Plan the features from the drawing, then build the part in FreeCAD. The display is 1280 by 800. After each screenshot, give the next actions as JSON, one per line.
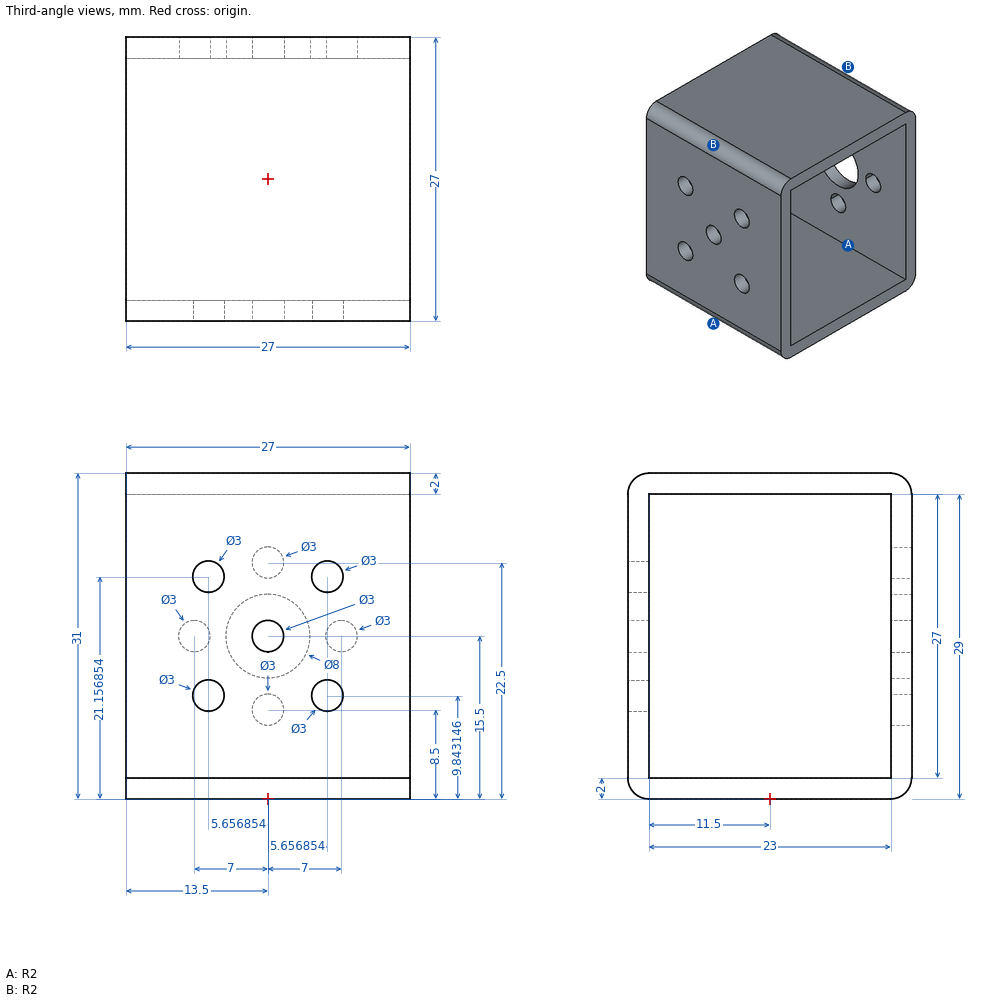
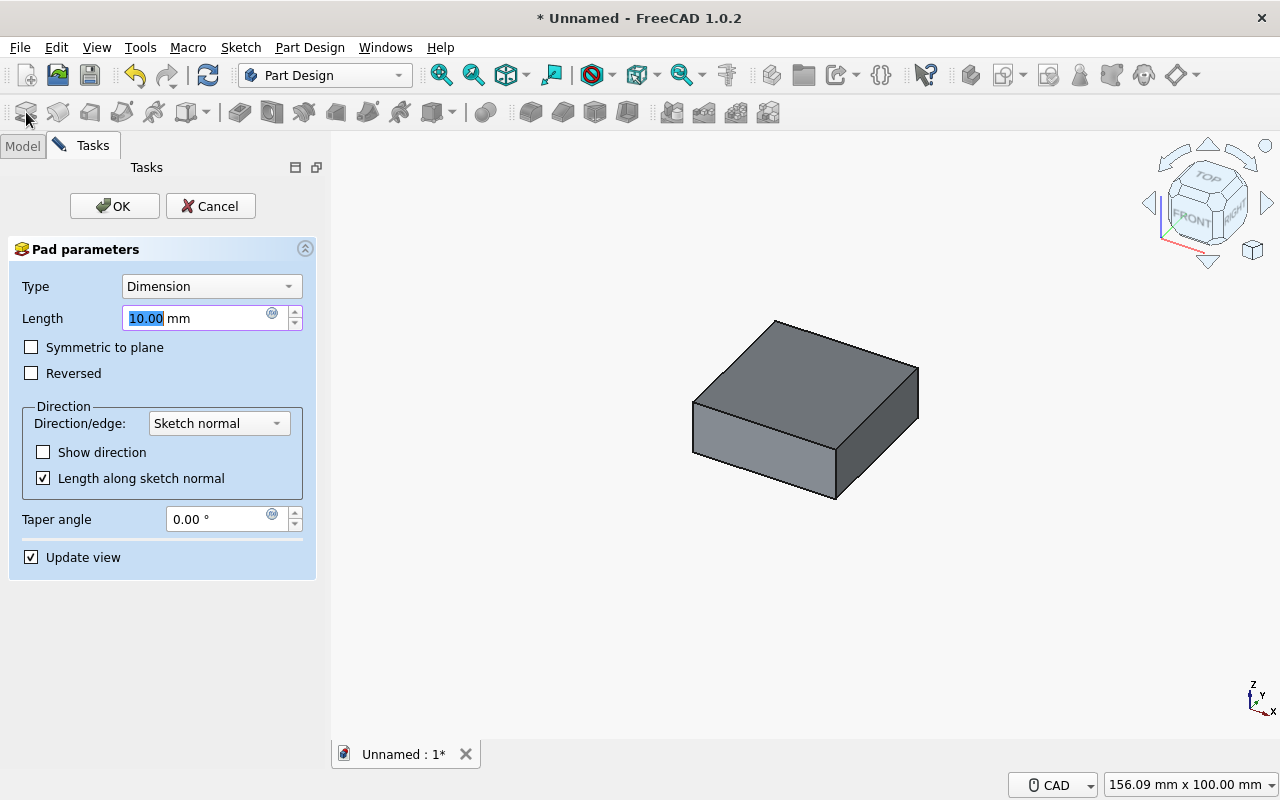
{"action": "type", "text": "29"}
{"action": "key", "text": "Tab"}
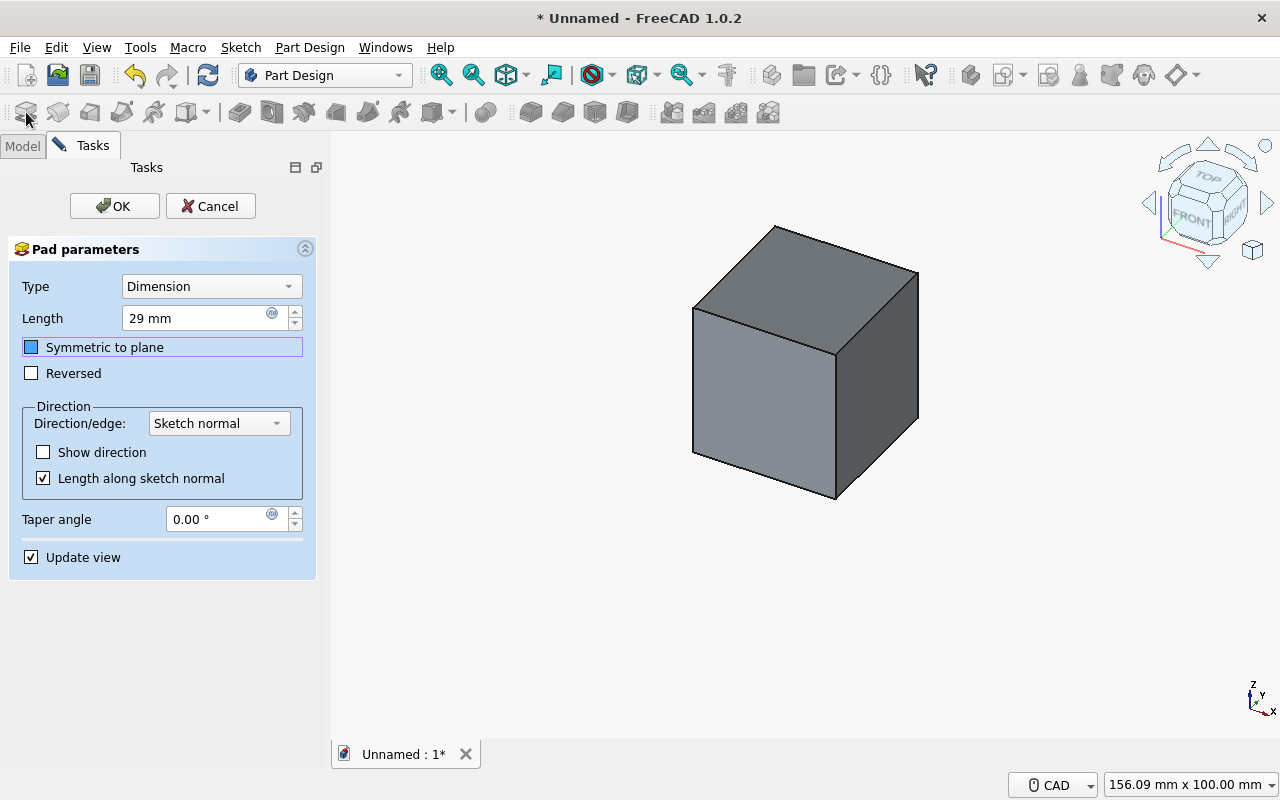
{"action": "left_click", "coordinate": [115, 206]}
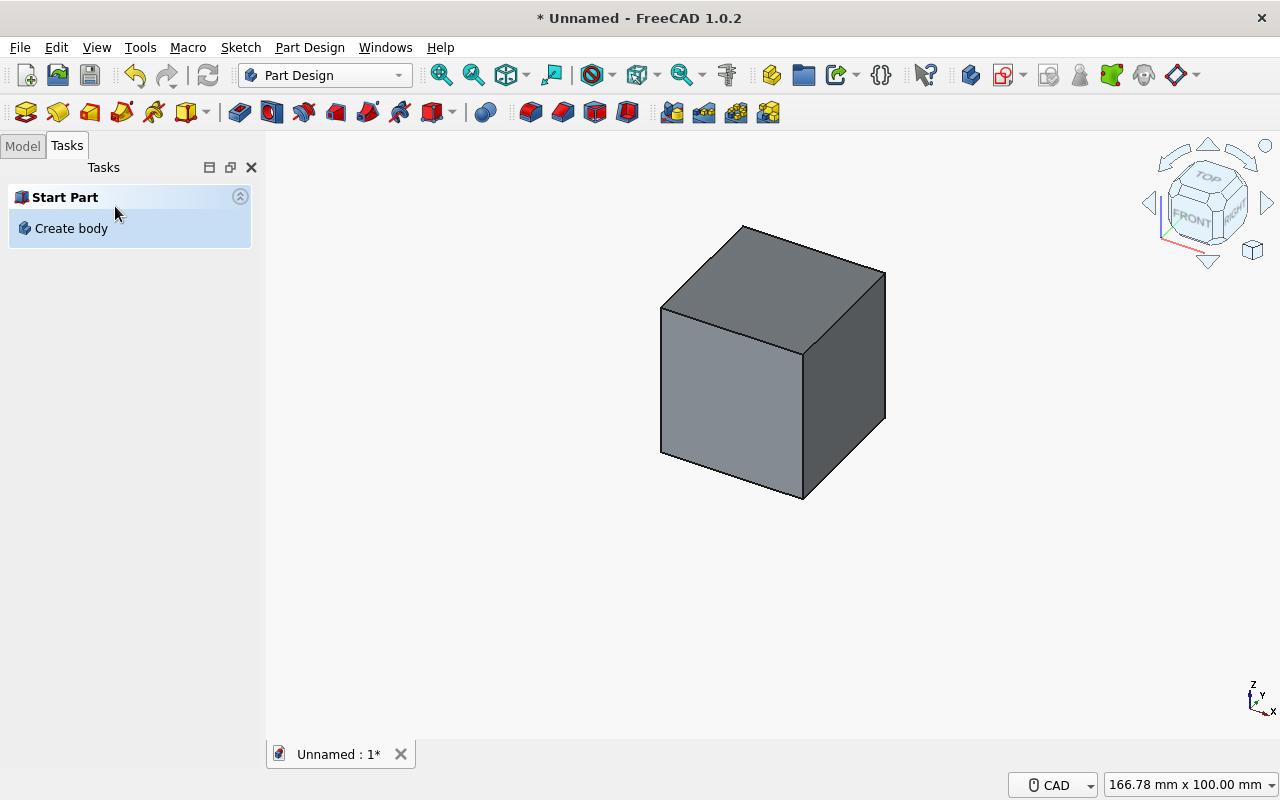
{"action": "left_click", "coordinate": [442, 76]}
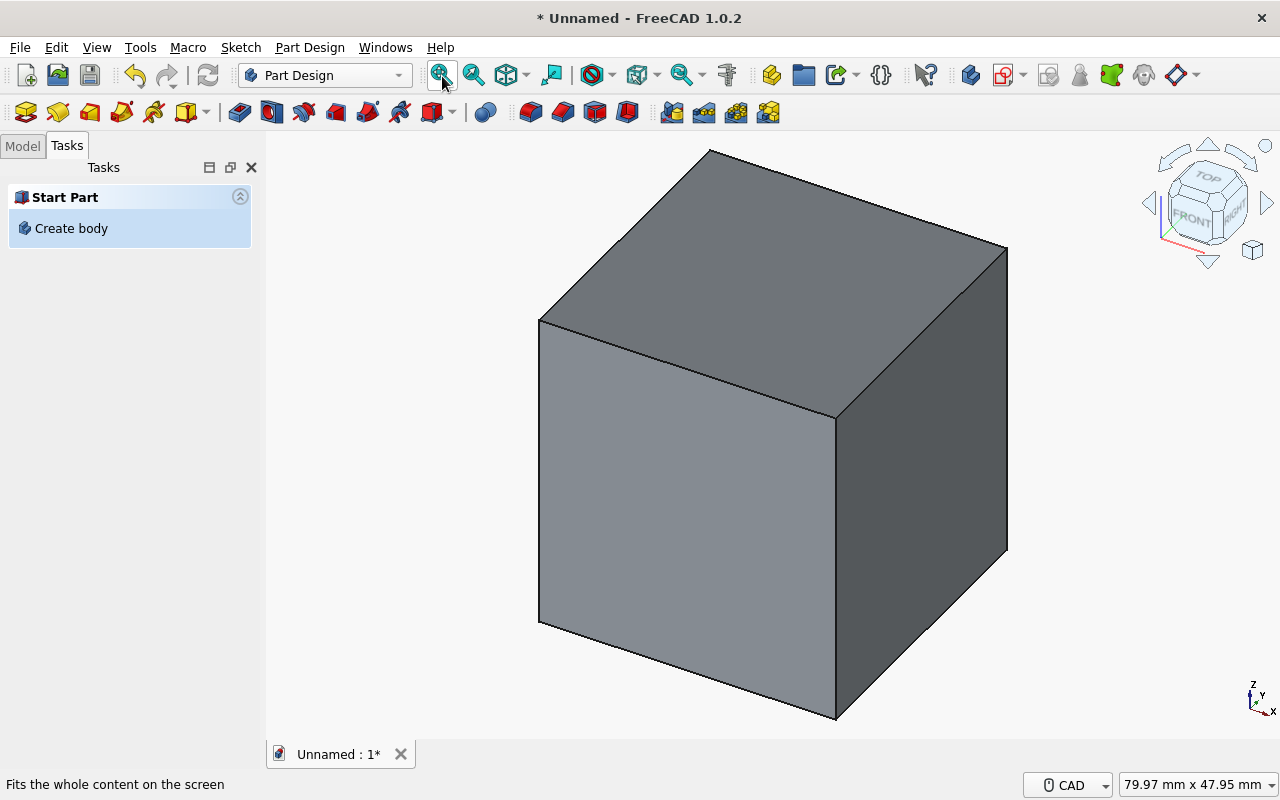
{"action": "left_click", "coordinate": [921, 483]}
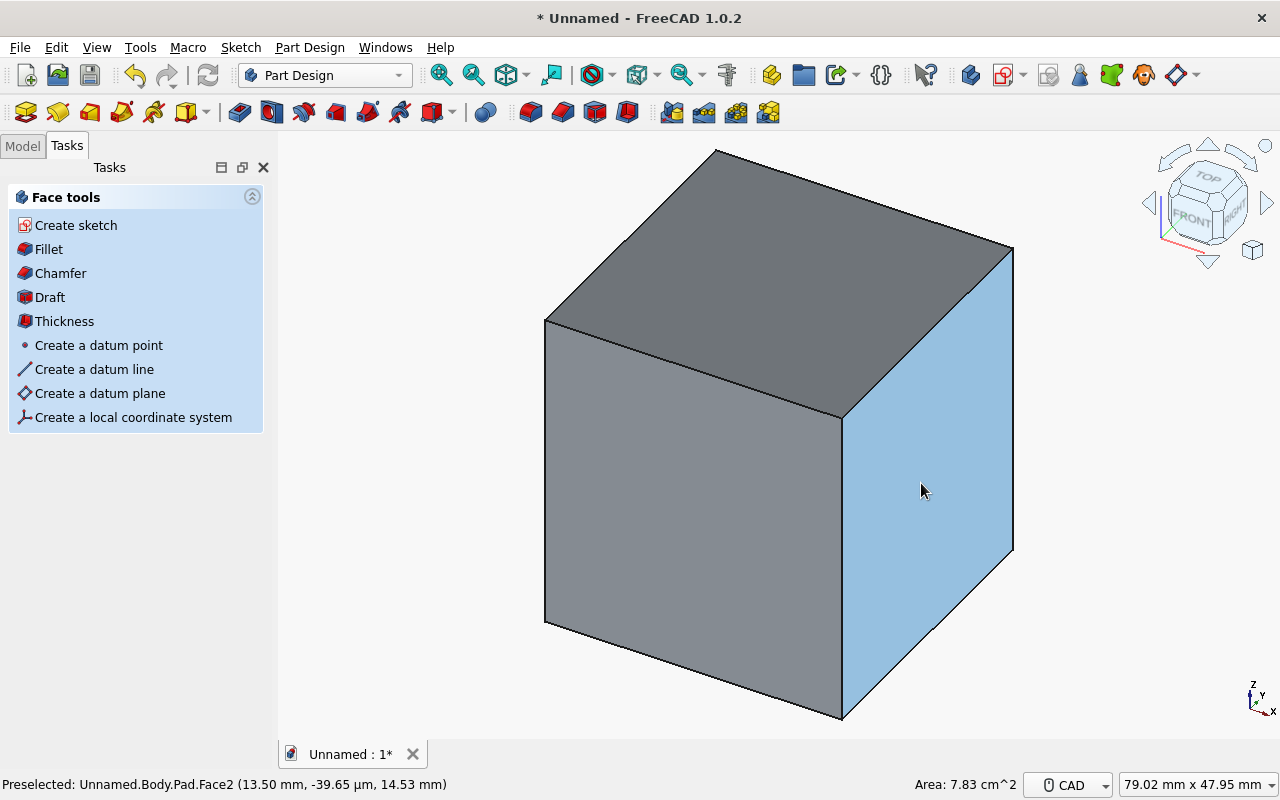
{"action": "left_click", "coordinate": [1004, 76]}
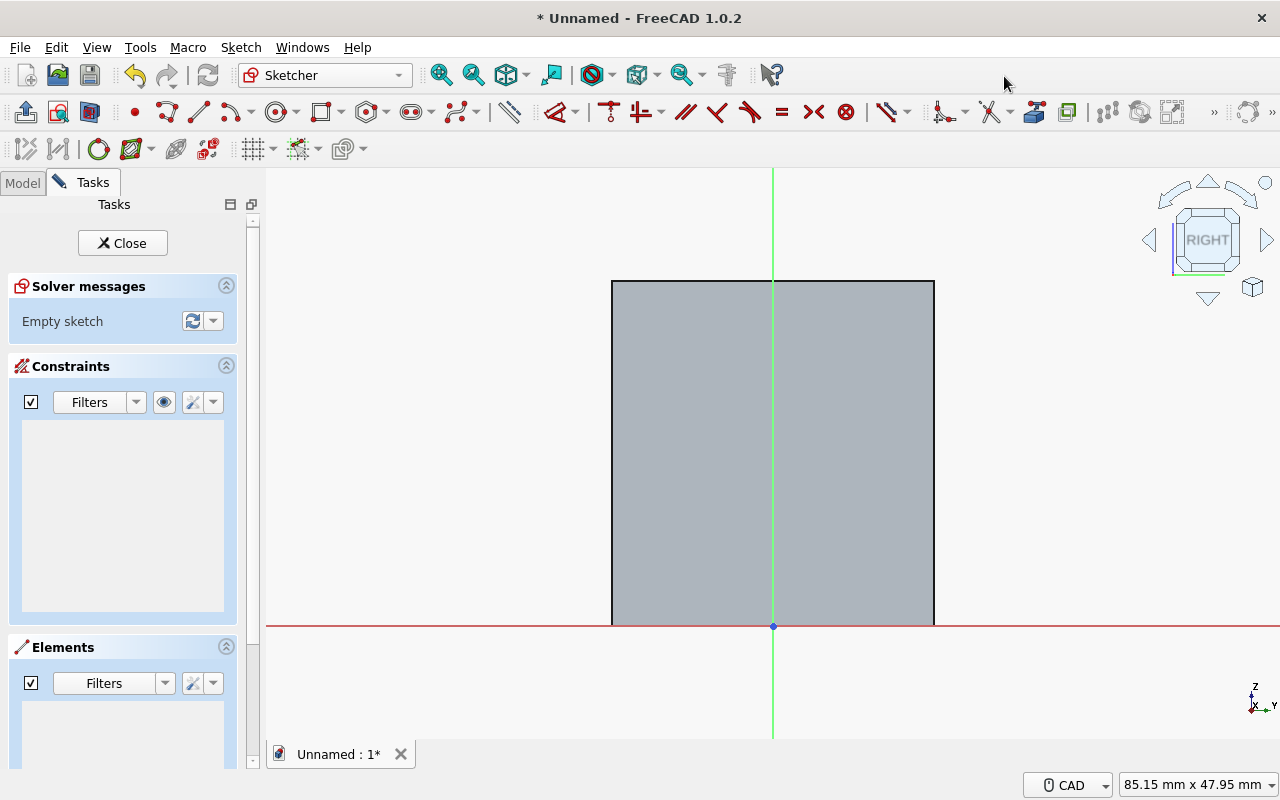
{"action": "left_click", "coordinate": [322, 112]}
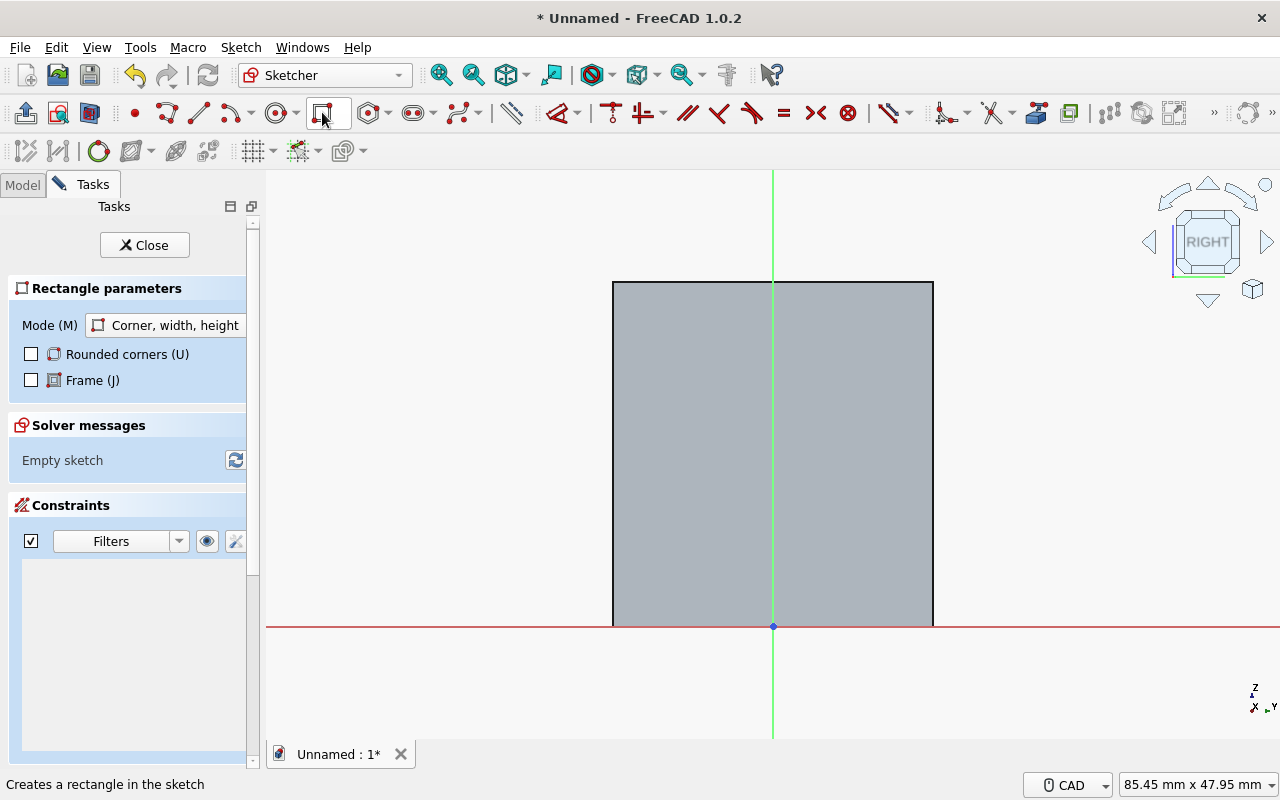
{"action": "left_click", "coordinate": [637, 282]}
{"action": "mouse_move", "coordinate": [909, 603]}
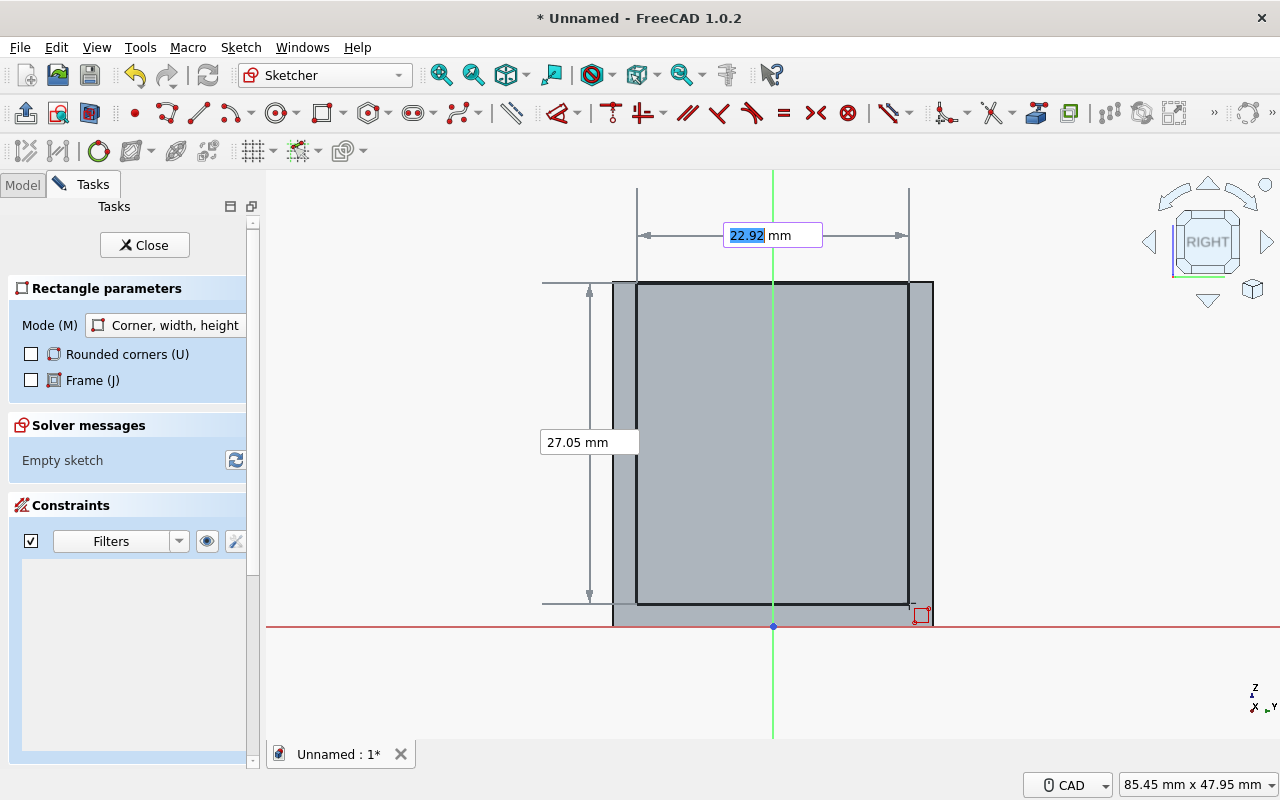
{"action": "type", "text": "23"}
{"action": "key", "text": "Tab"}
{"action": "type", "text": "27"}
{"action": "key", "text": "Return"}
{"action": "key", "text": "Escape"}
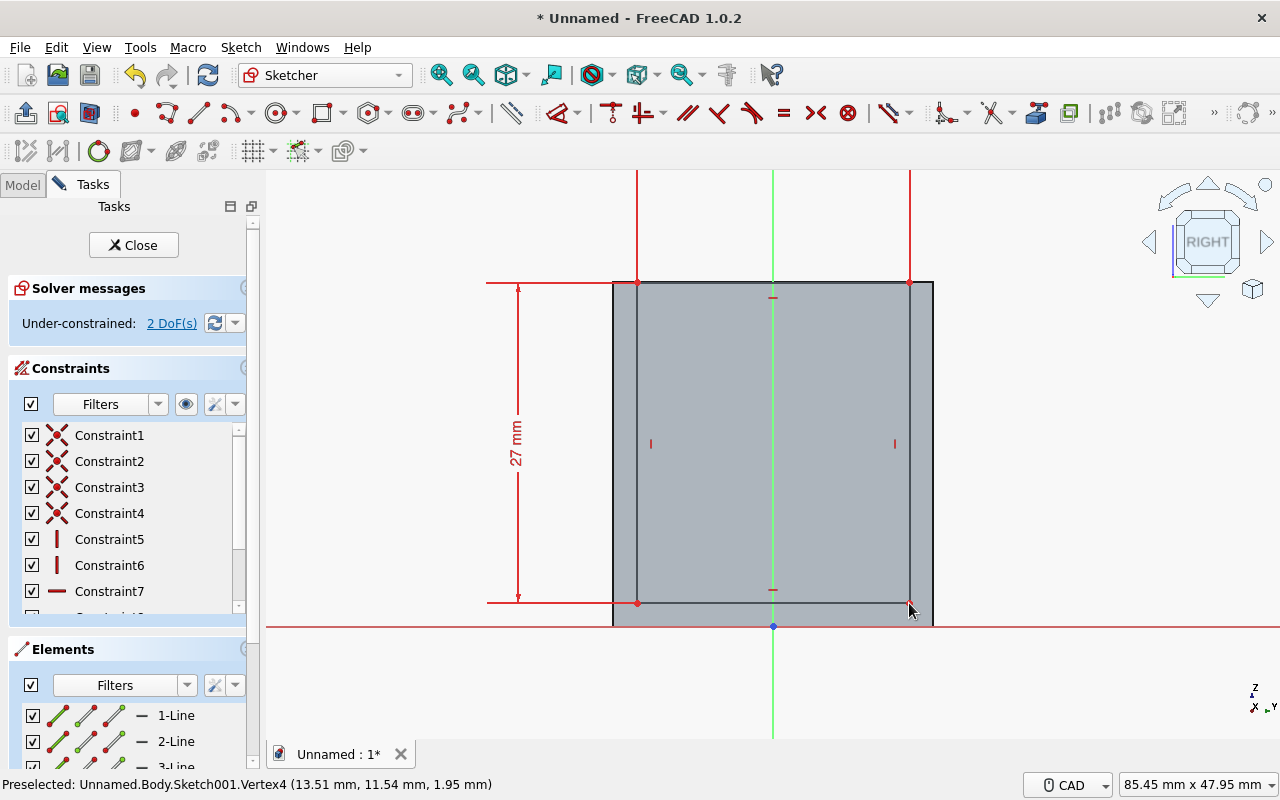
{"action": "left_click", "coordinate": [558, 114]}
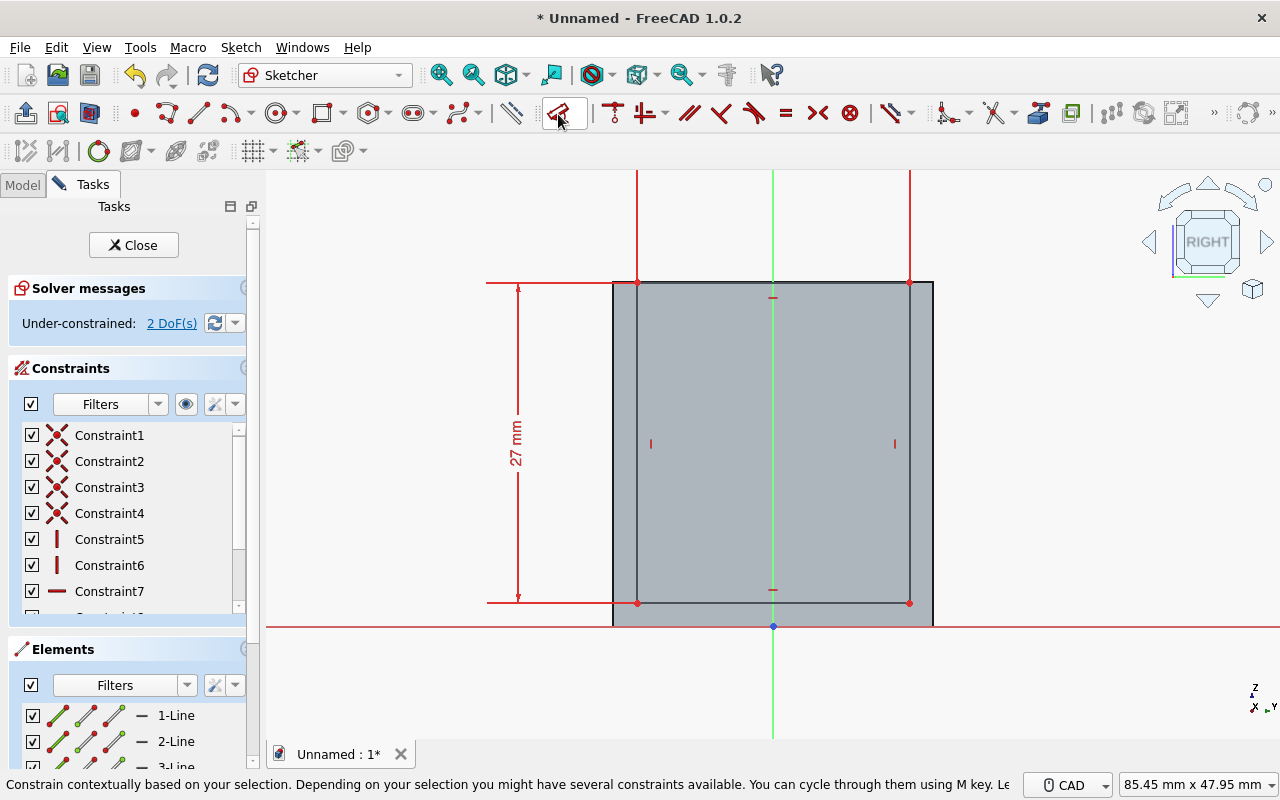
{"action": "scroll", "coordinate": [637, 603], "scroll_direction": "up", "scroll_amount": 3}